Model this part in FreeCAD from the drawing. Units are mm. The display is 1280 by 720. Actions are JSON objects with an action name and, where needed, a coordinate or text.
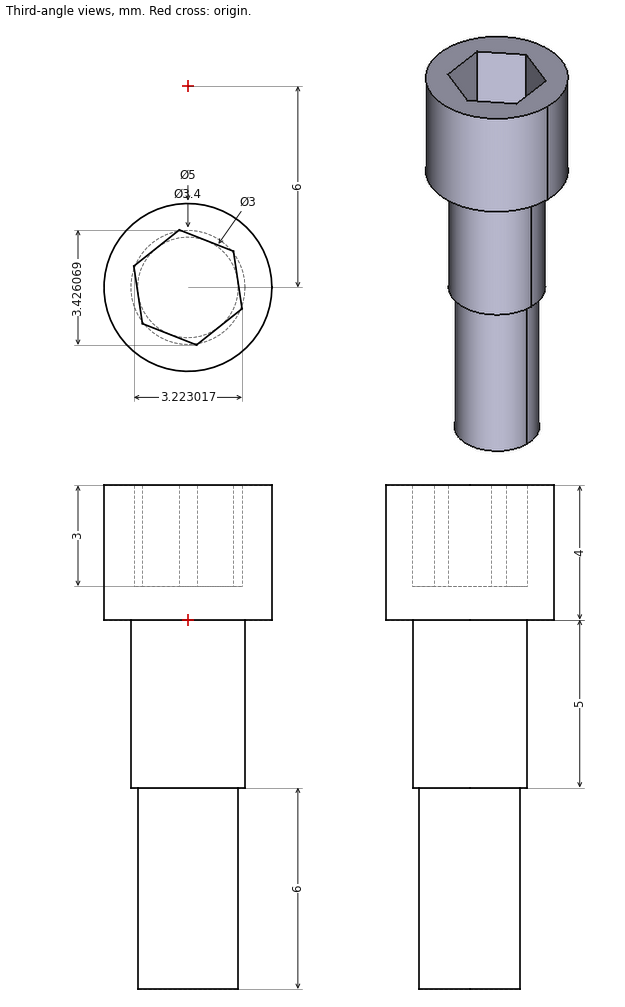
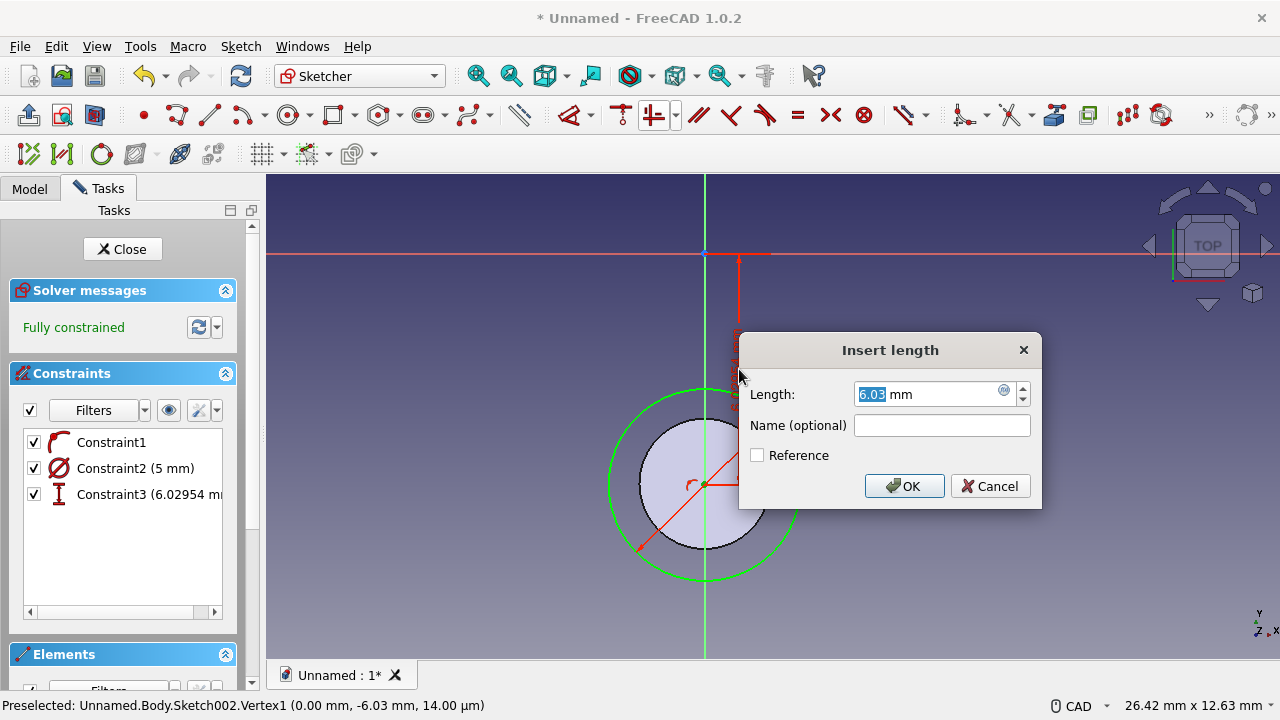
{"action": "type", "text": "6"}
{"action": "key", "text": "Return"}
{"action": "key", "text": "Escape"}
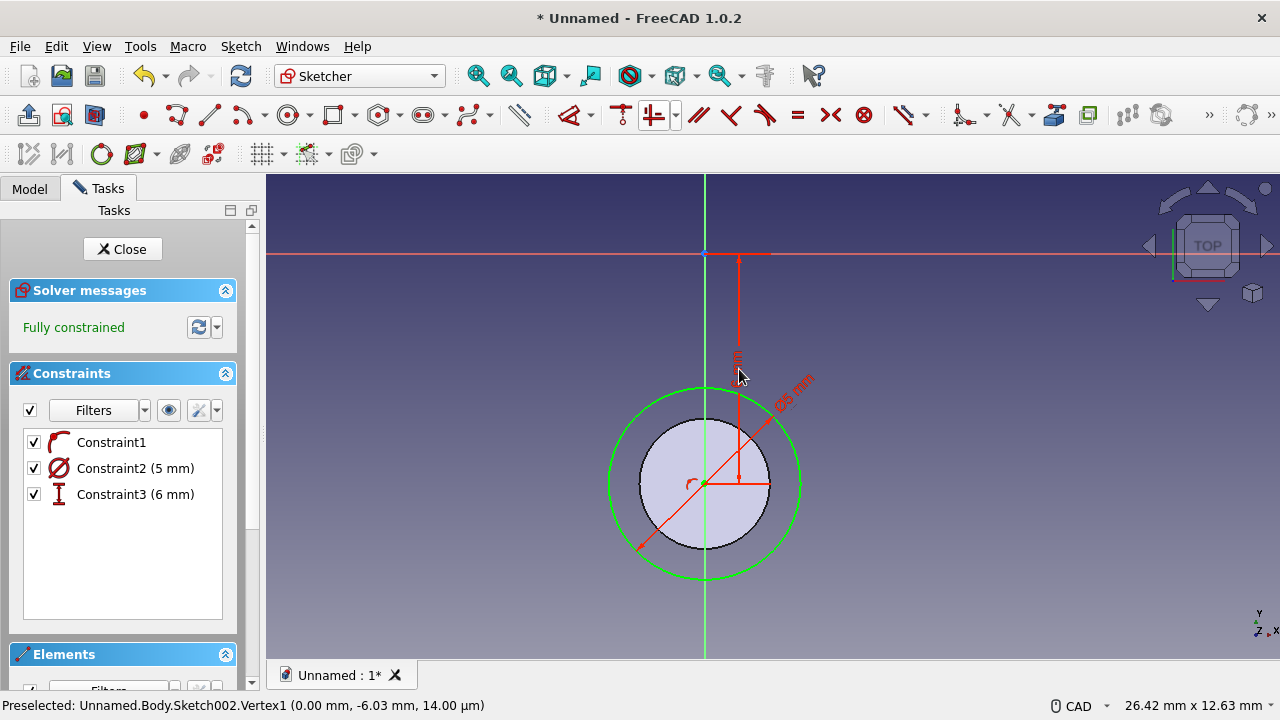
{"action": "left_click", "coordinate": [123, 249]}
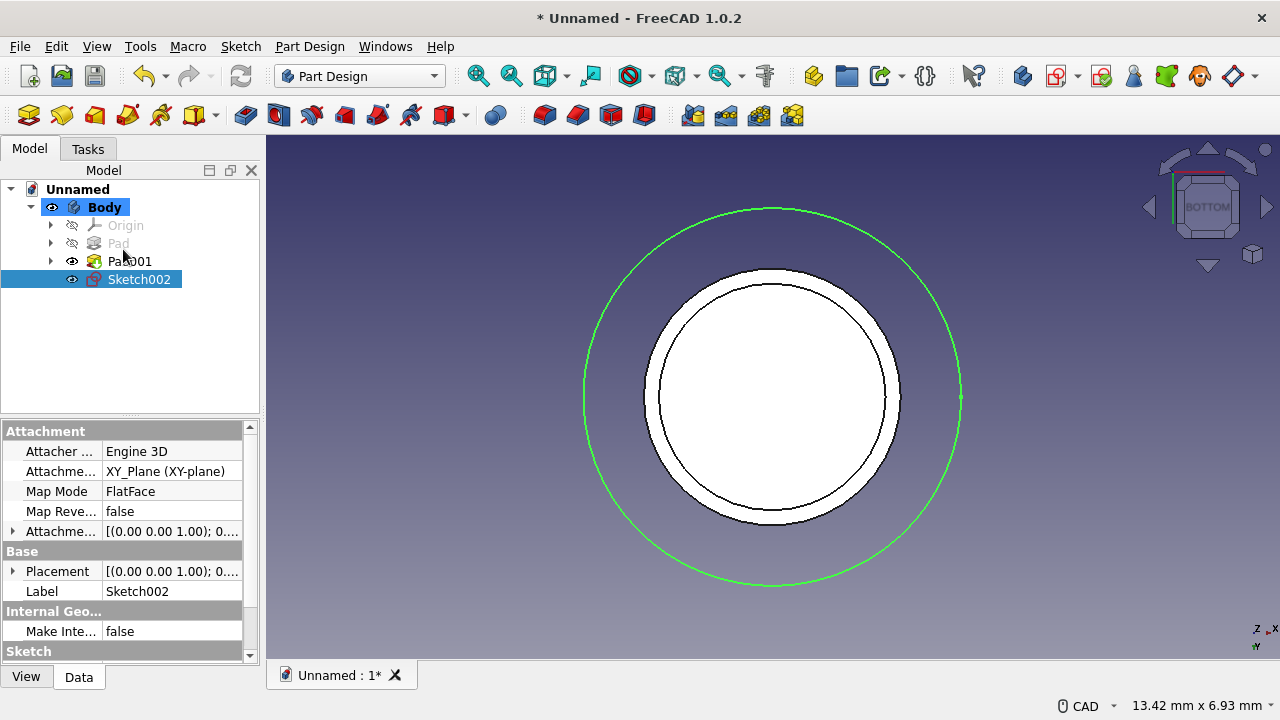
{"action": "left_click", "coordinate": [29, 116]}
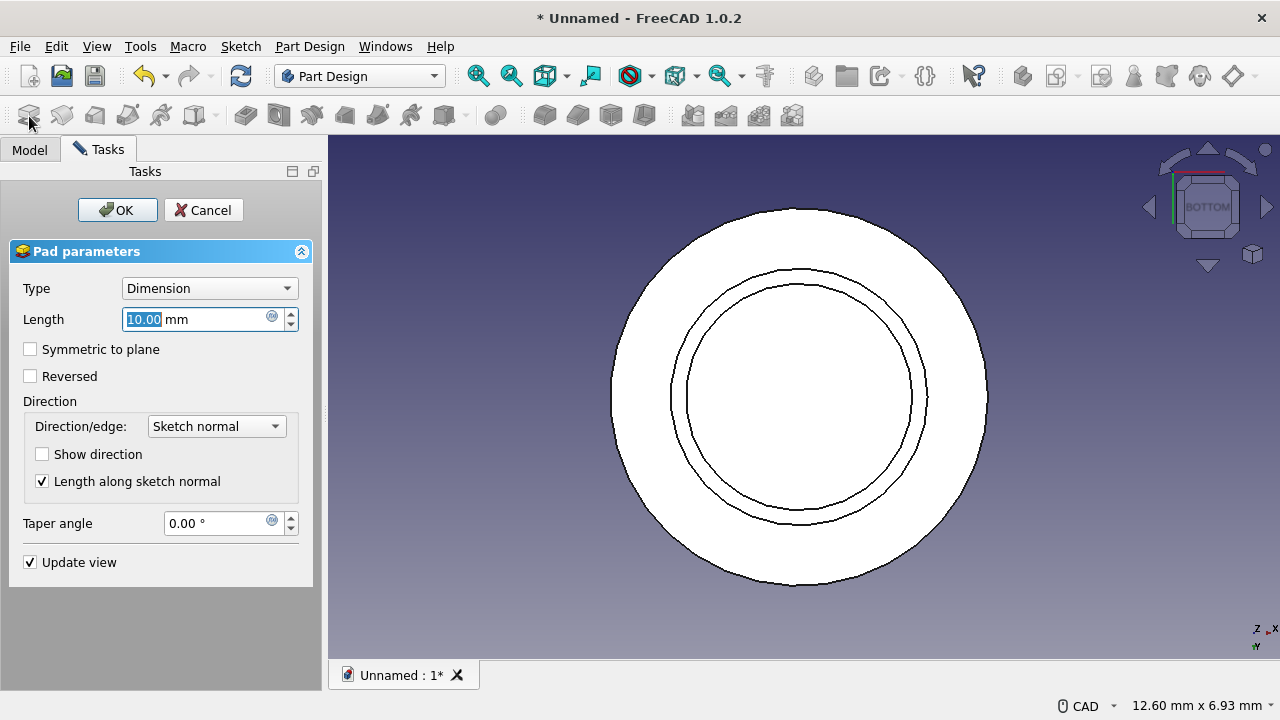
{"action": "type", "text": "4"}
{"action": "key", "text": "Tab"}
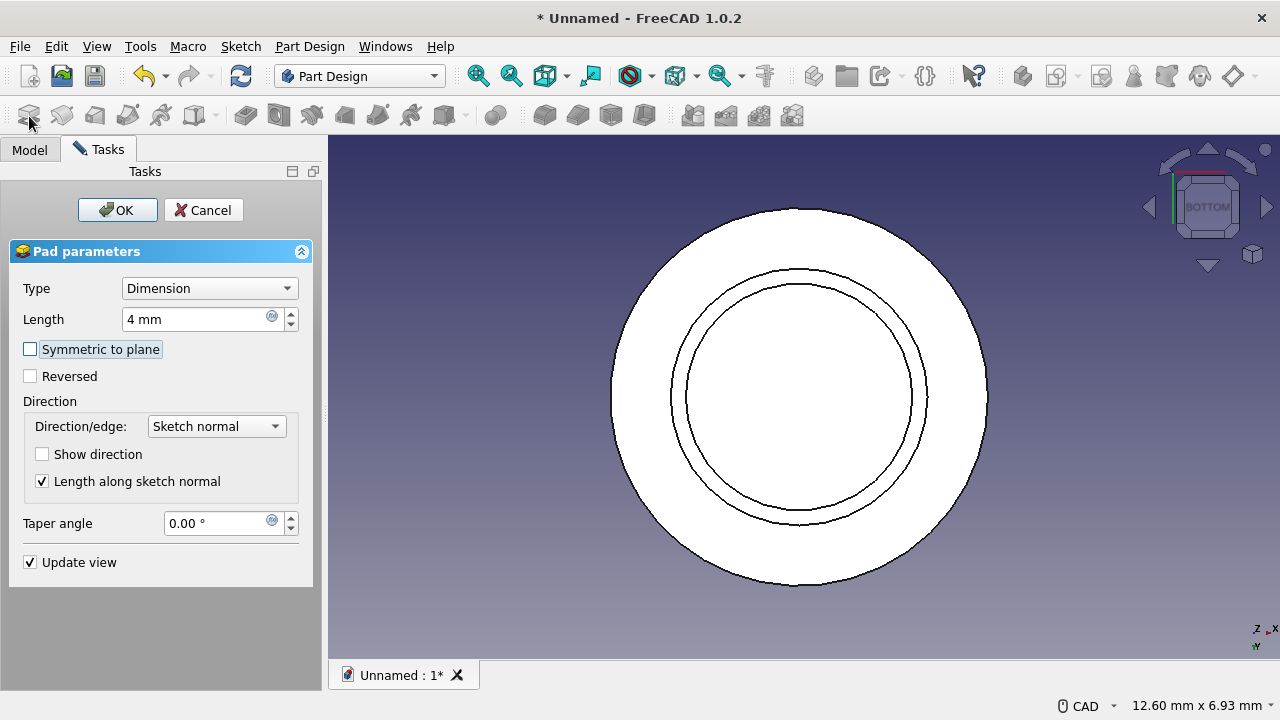
{"action": "left_click", "coordinate": [118, 210]}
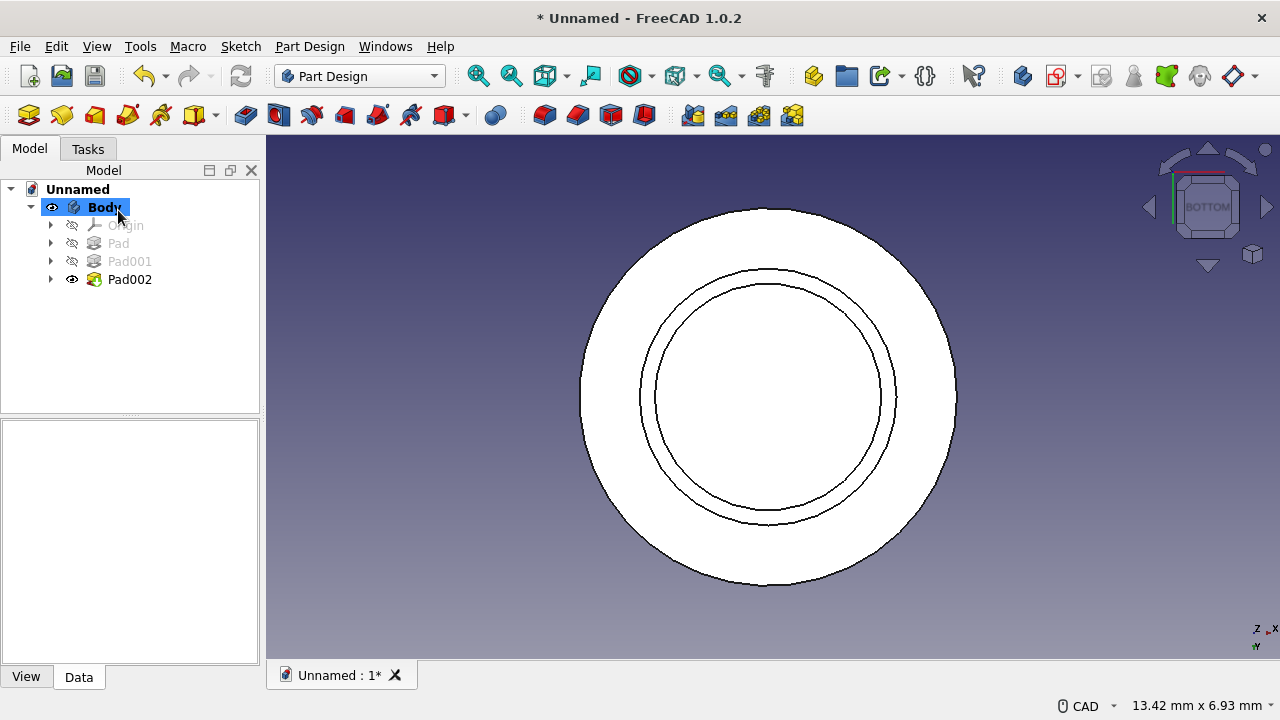
{"action": "key", "text": "0"}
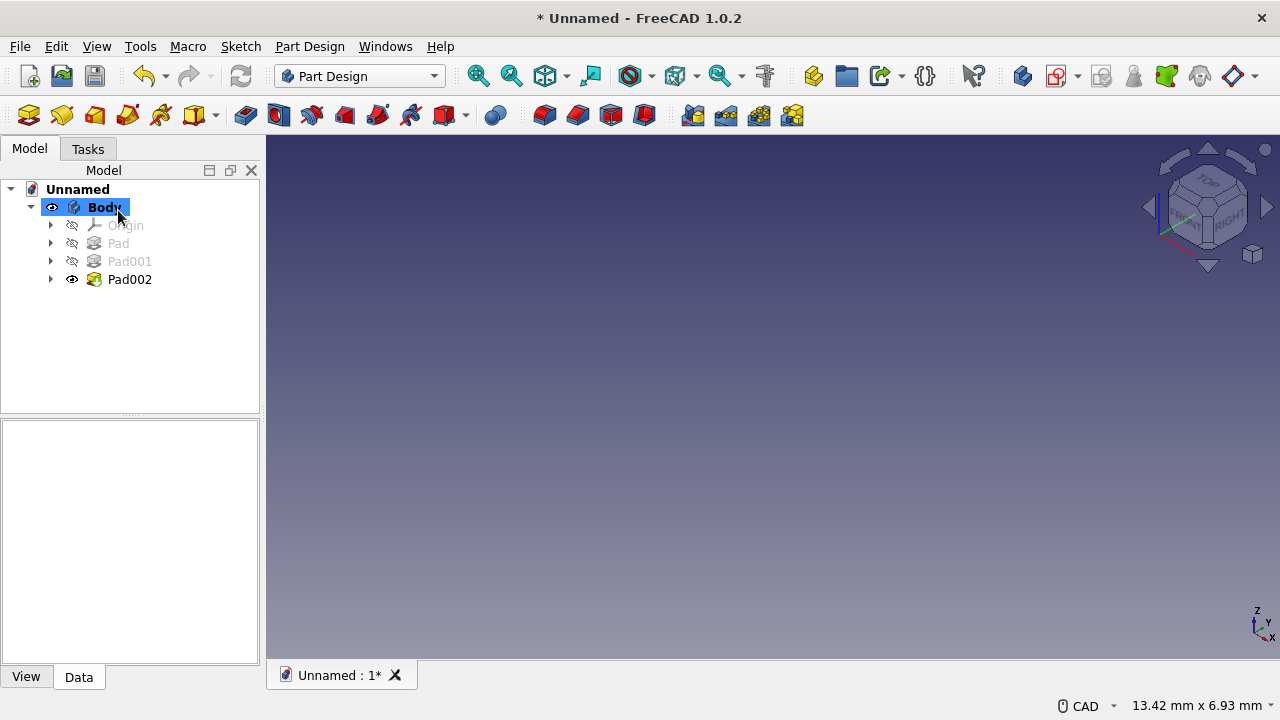
{"action": "key", "text": "v f"}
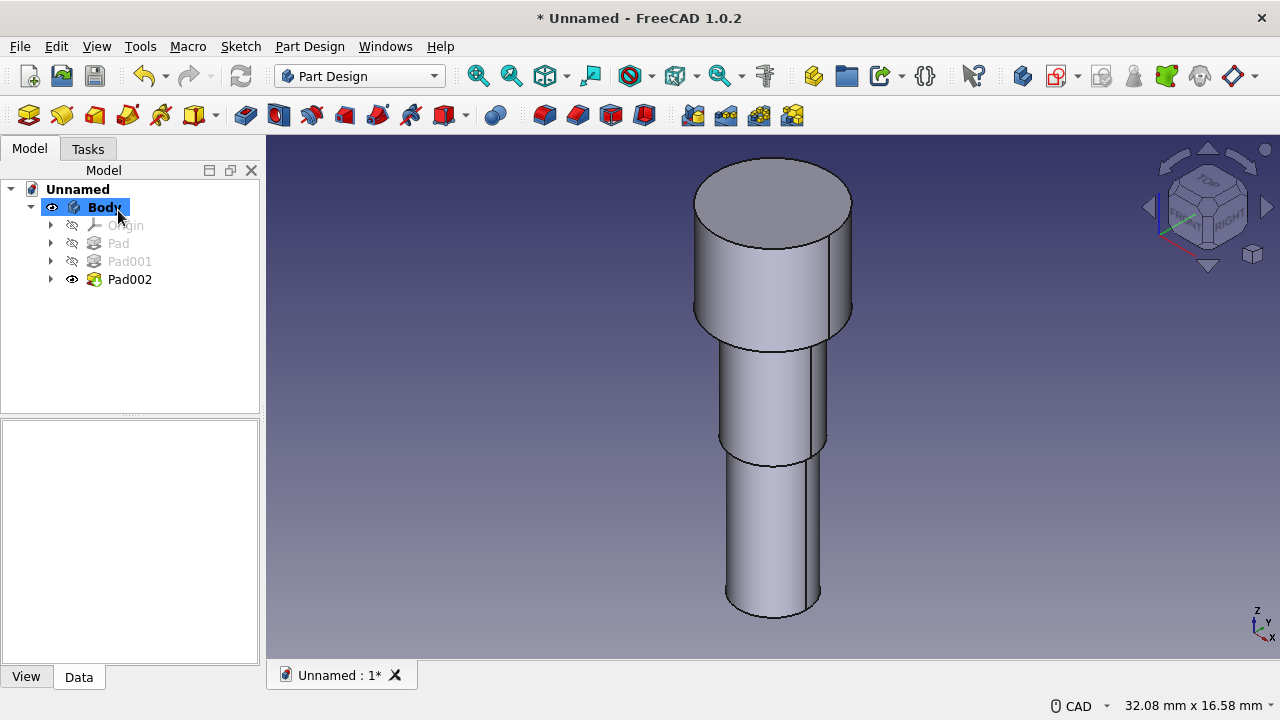
{"action": "left_click", "coordinate": [773, 202]}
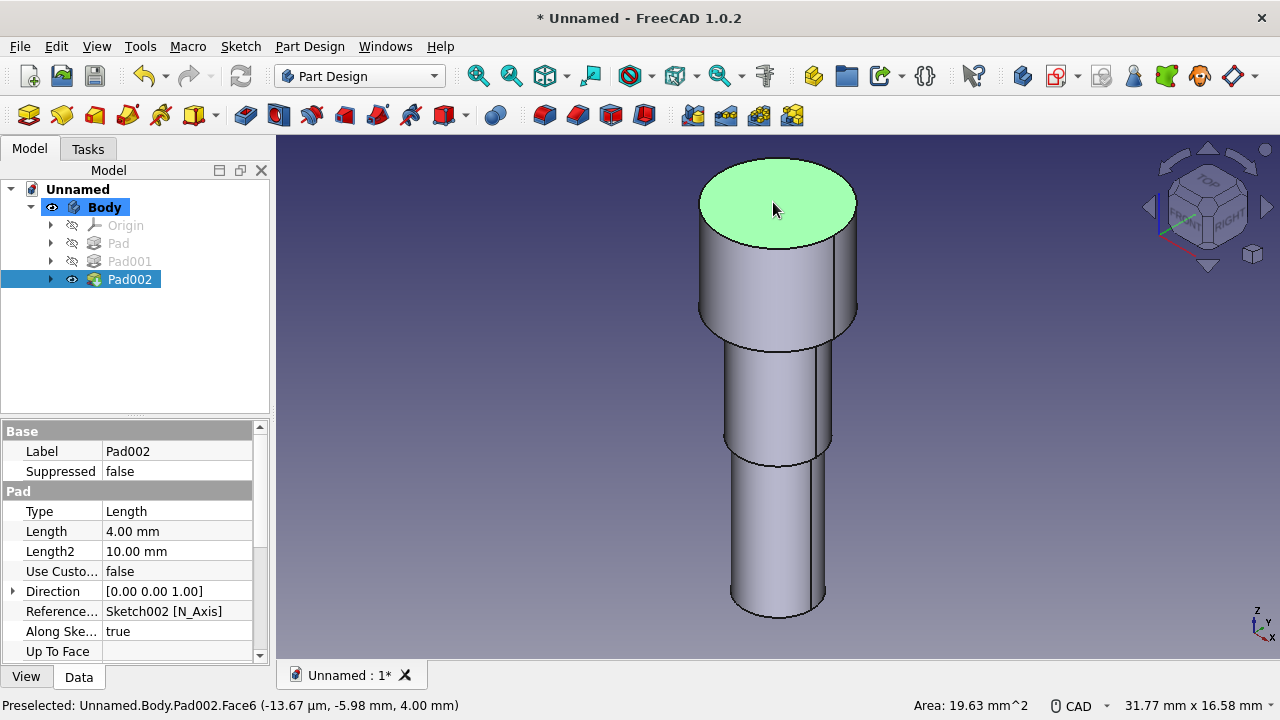
{"action": "left_click", "coordinate": [1056, 76]}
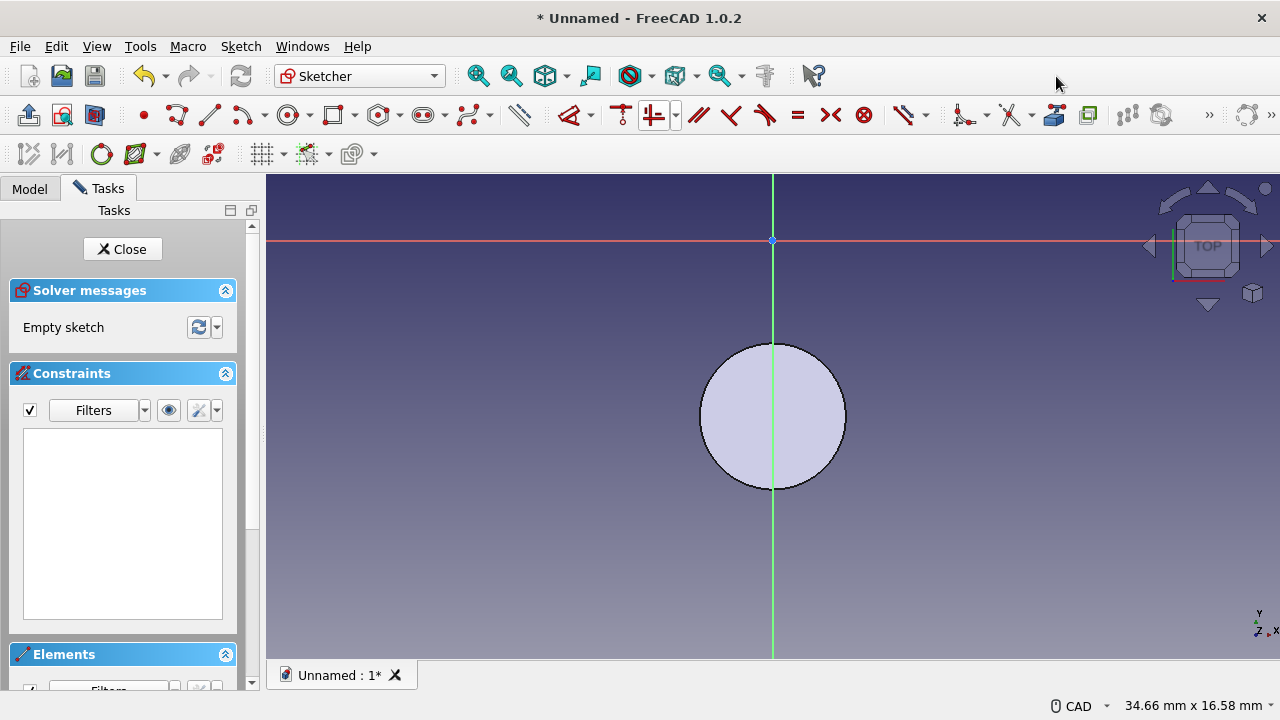
{"action": "key", "text": "g p 6"}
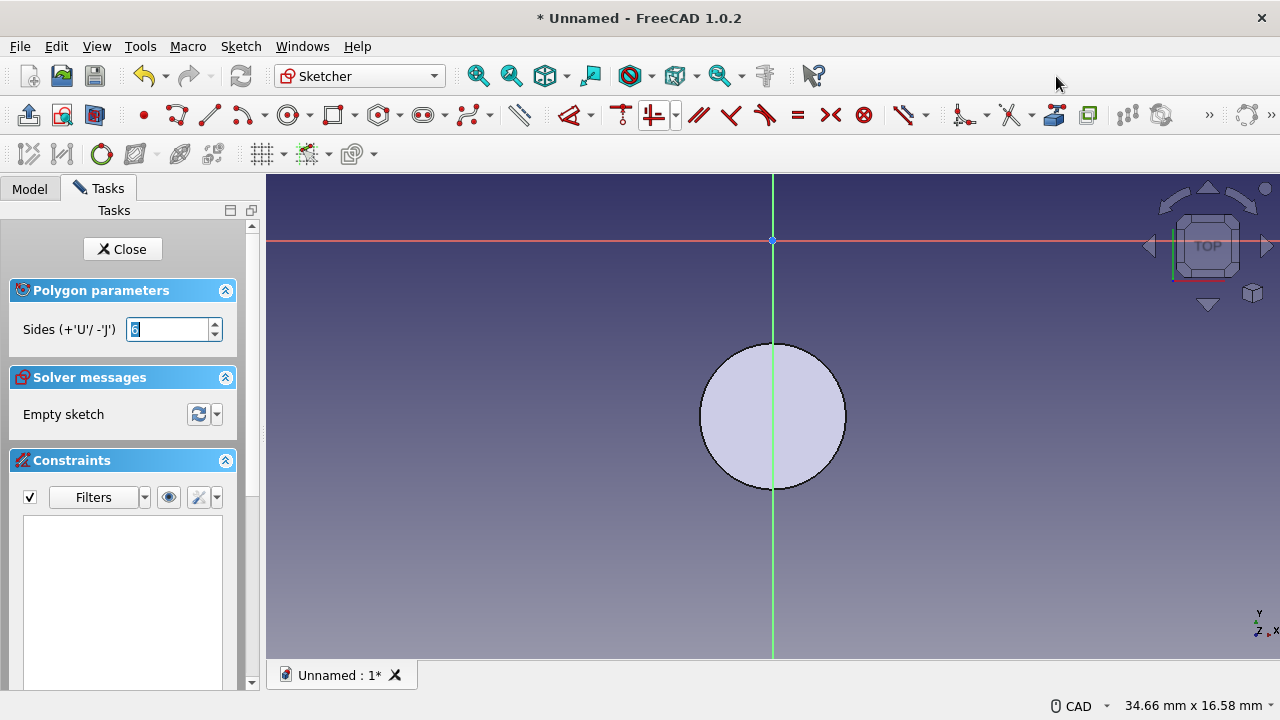
{"action": "left_click", "coordinate": [773, 416]}